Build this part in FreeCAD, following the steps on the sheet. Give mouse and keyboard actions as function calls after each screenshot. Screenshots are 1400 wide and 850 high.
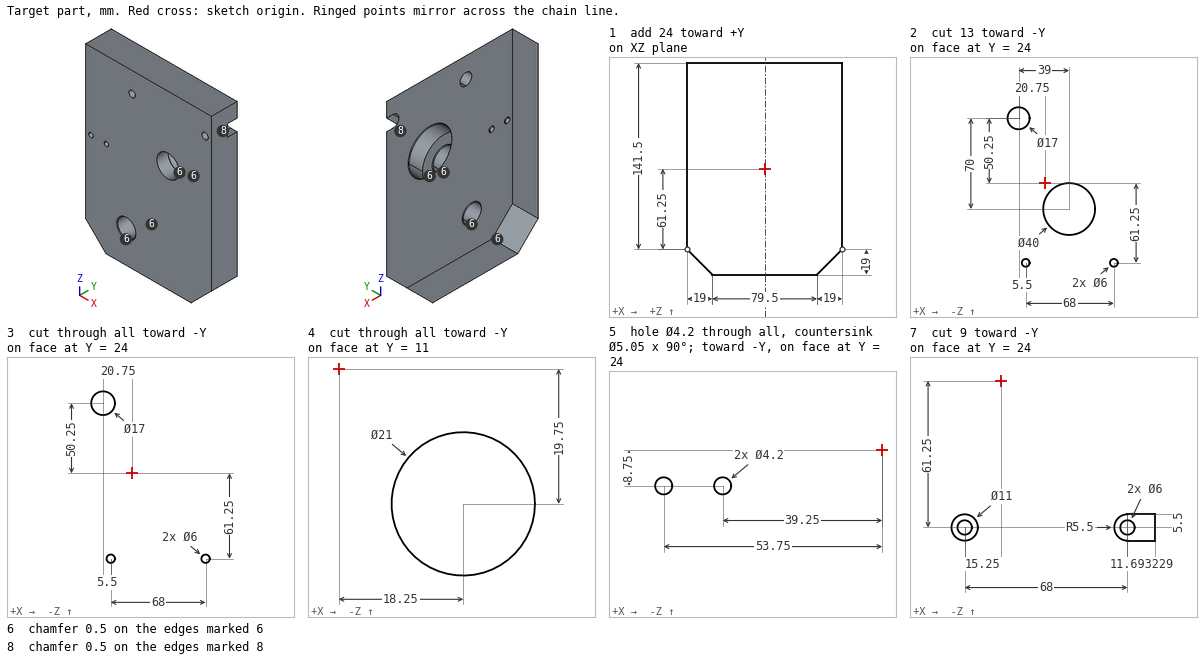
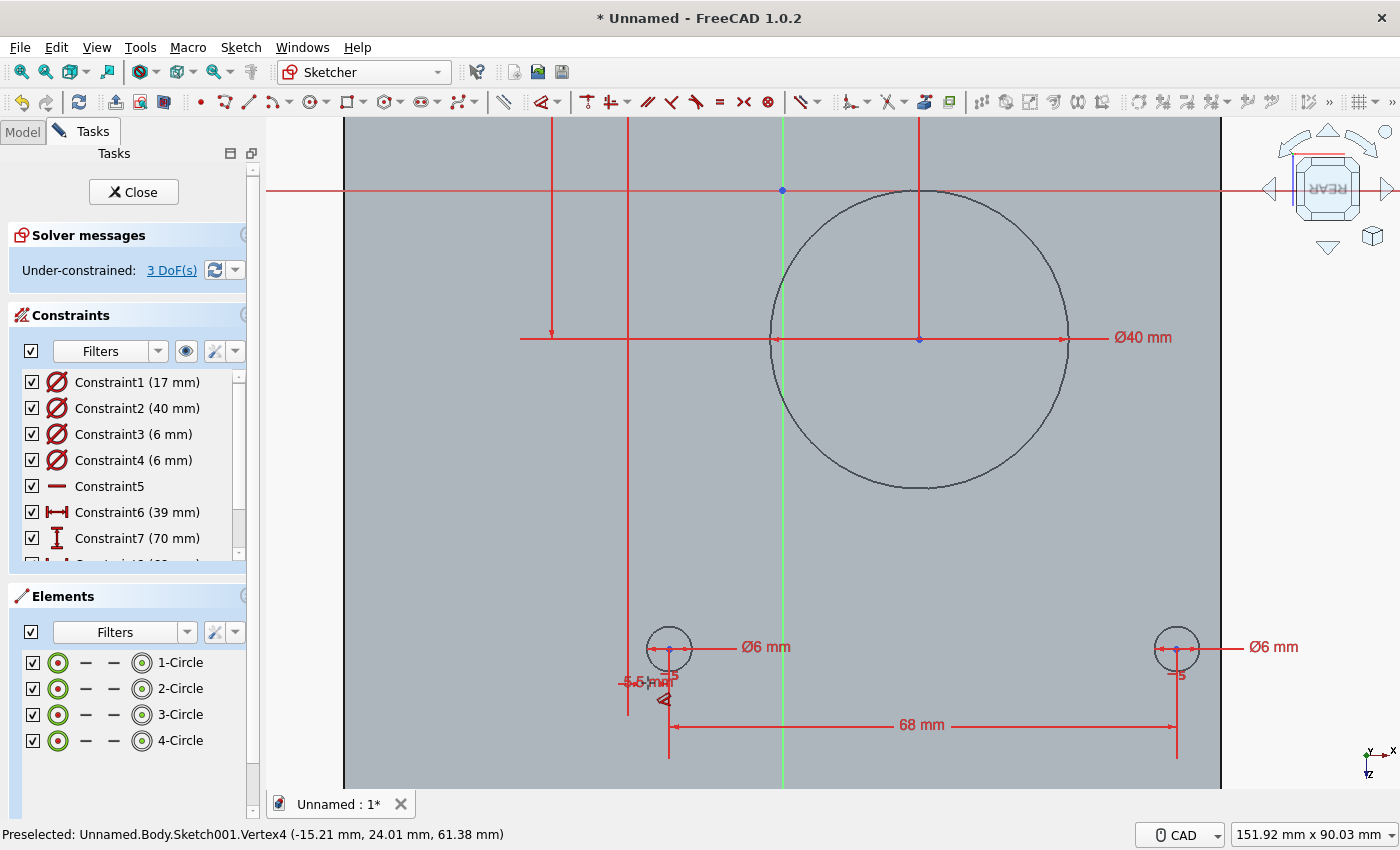
scroll(669, 650, down, 4)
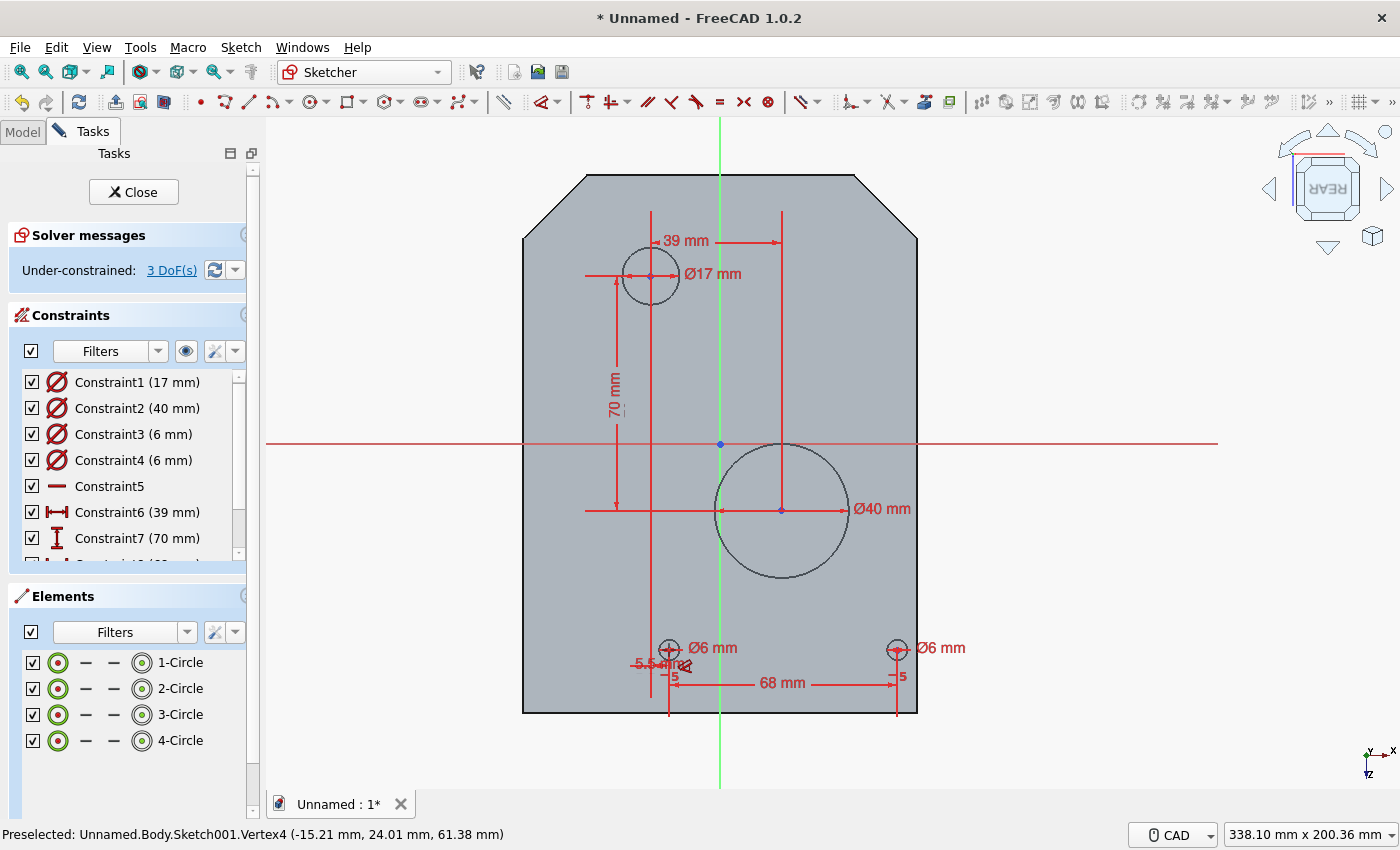
click(651, 276)
click(686, 478)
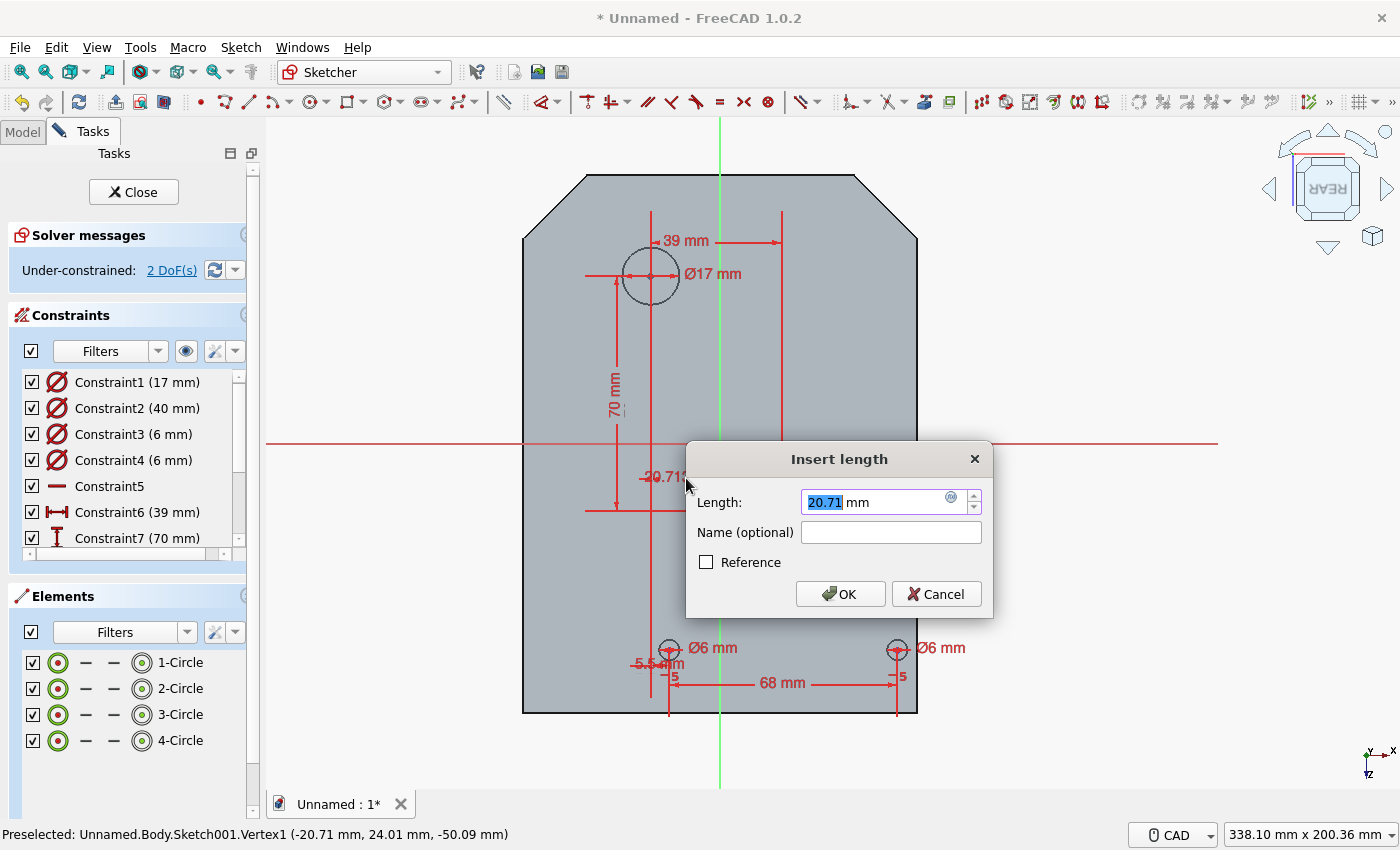
text(20.75)
key(Return)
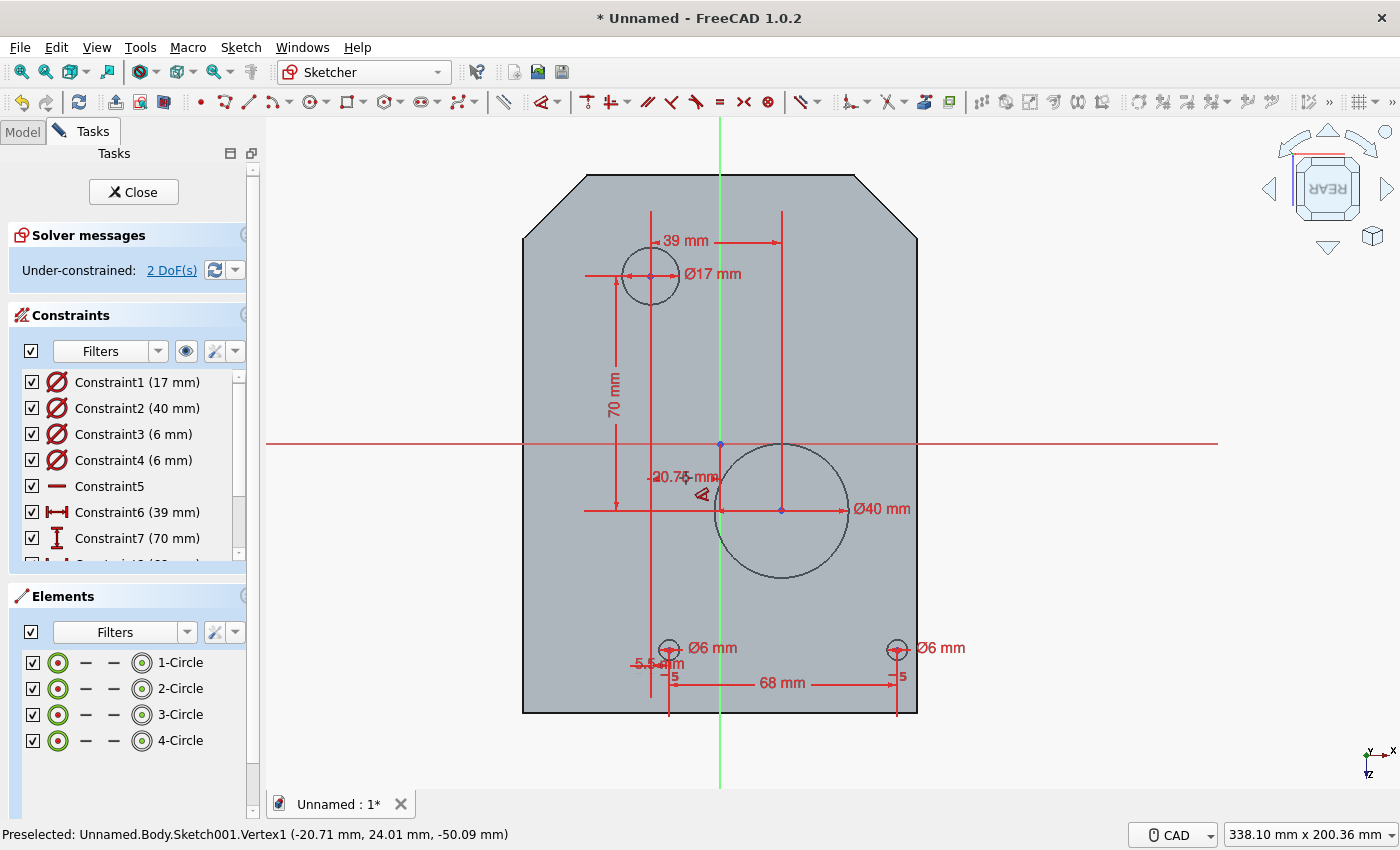
click(651, 276)
click(617, 360)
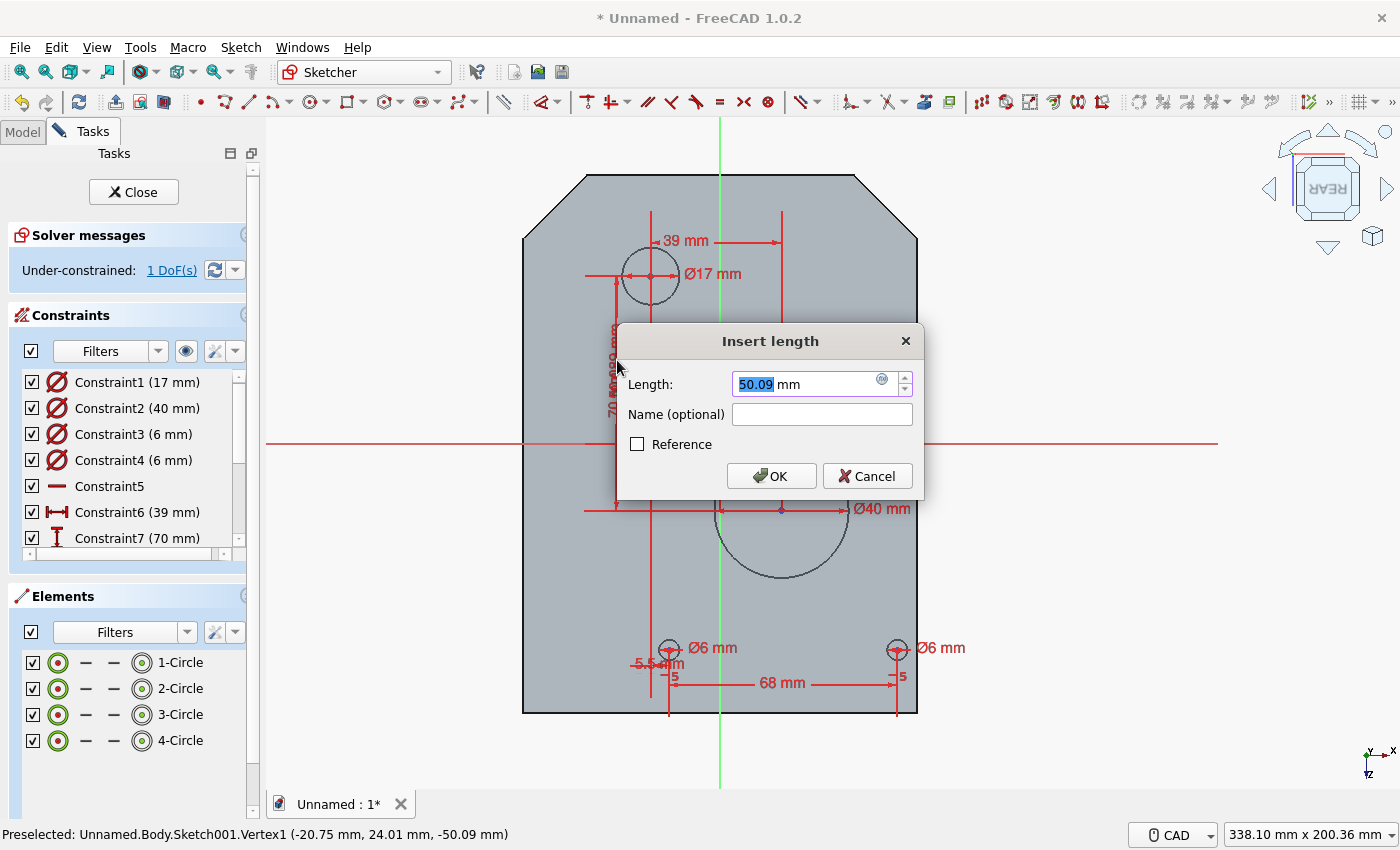
text(50.25)
key(Return)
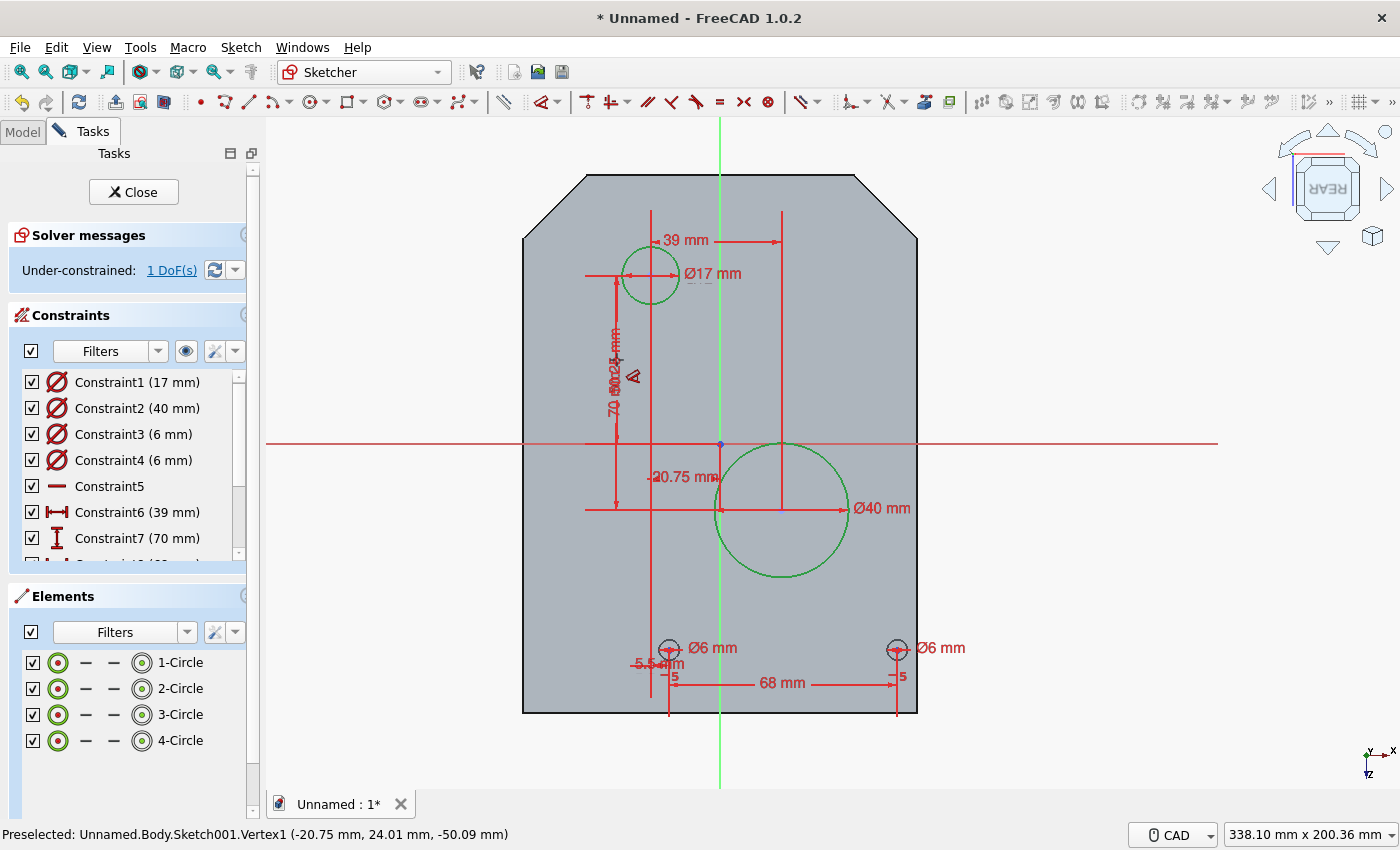
click(897, 650)
click(931, 547)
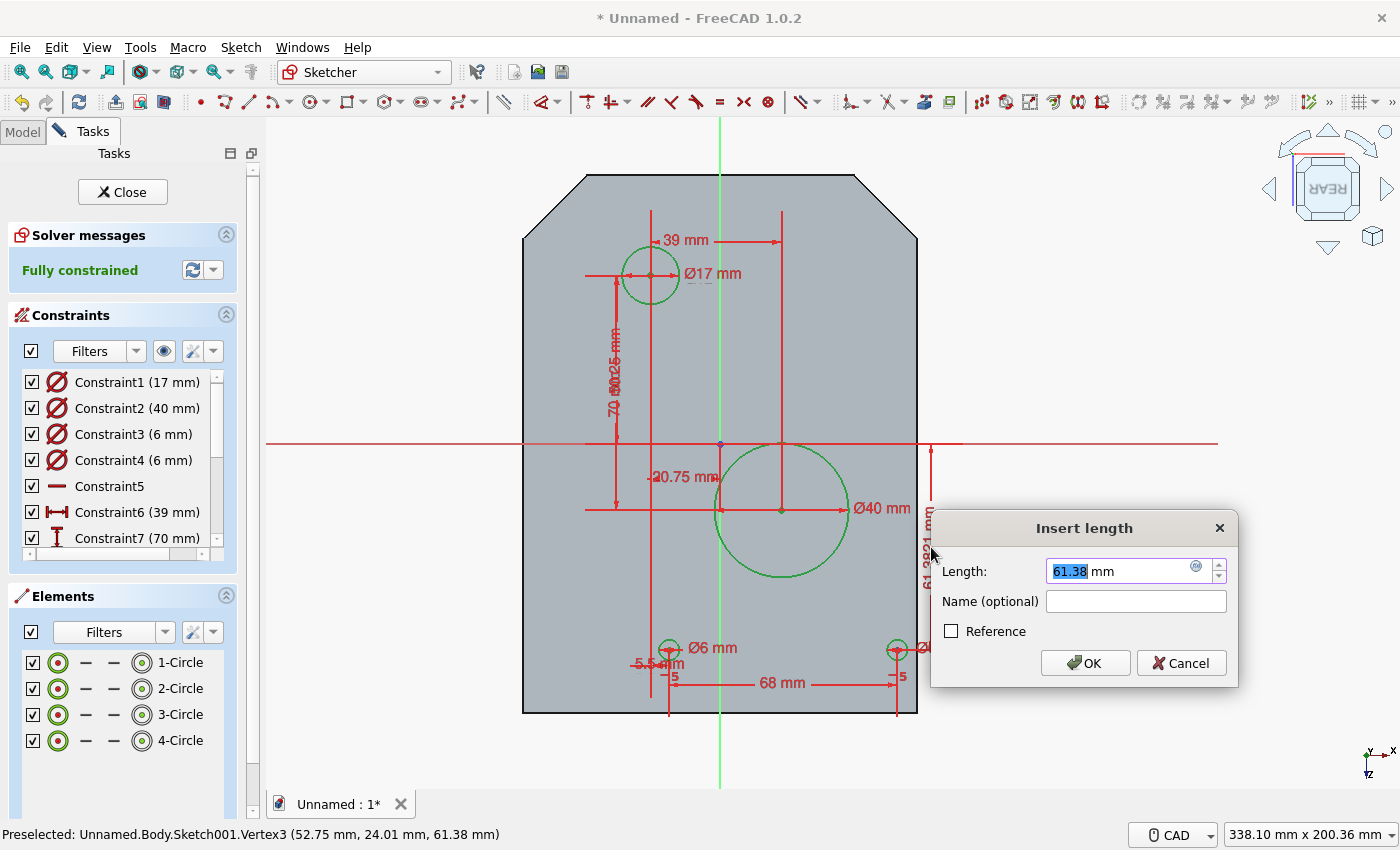
text(61.25)
key(Return)
key(Escape)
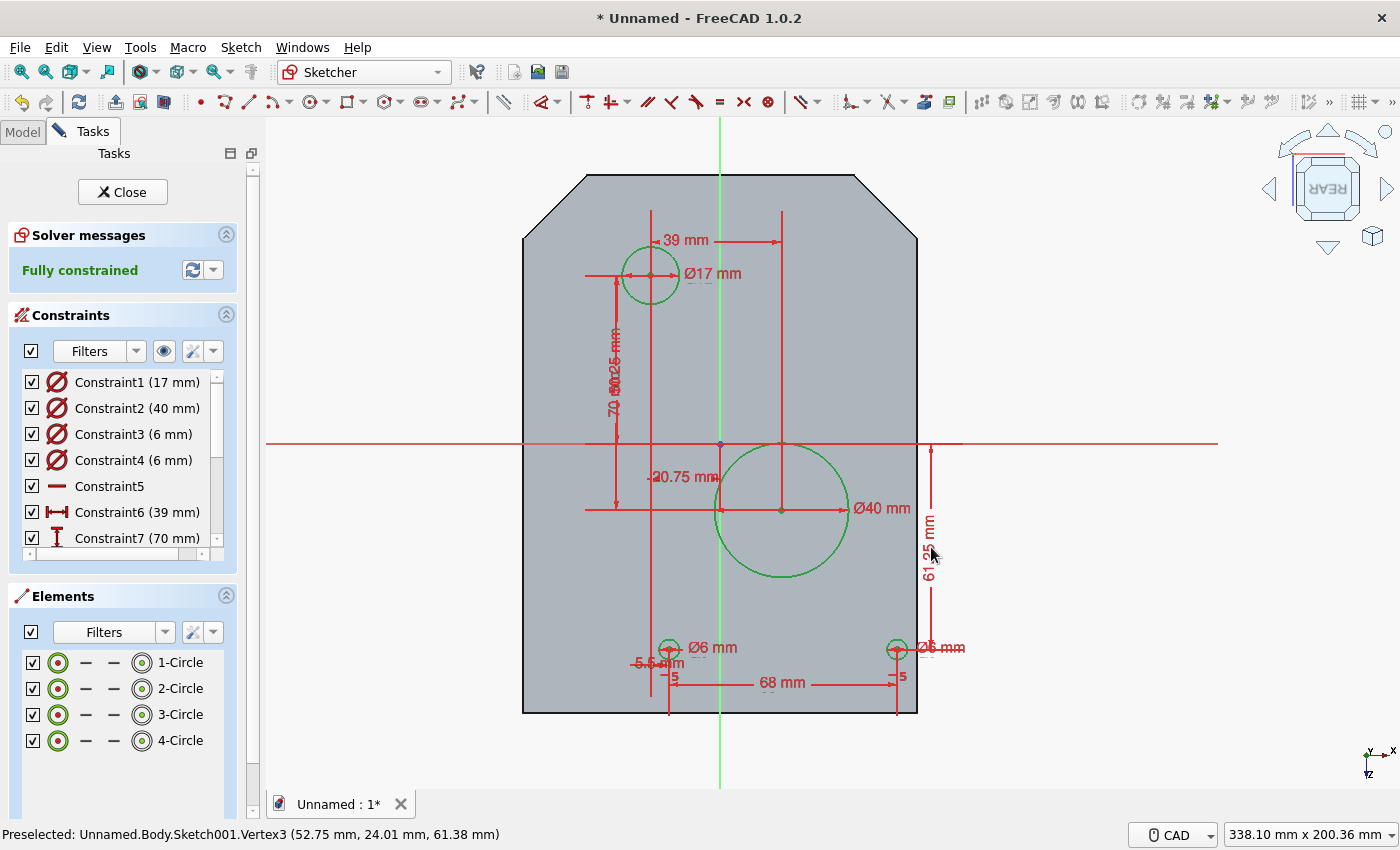
click(123, 192)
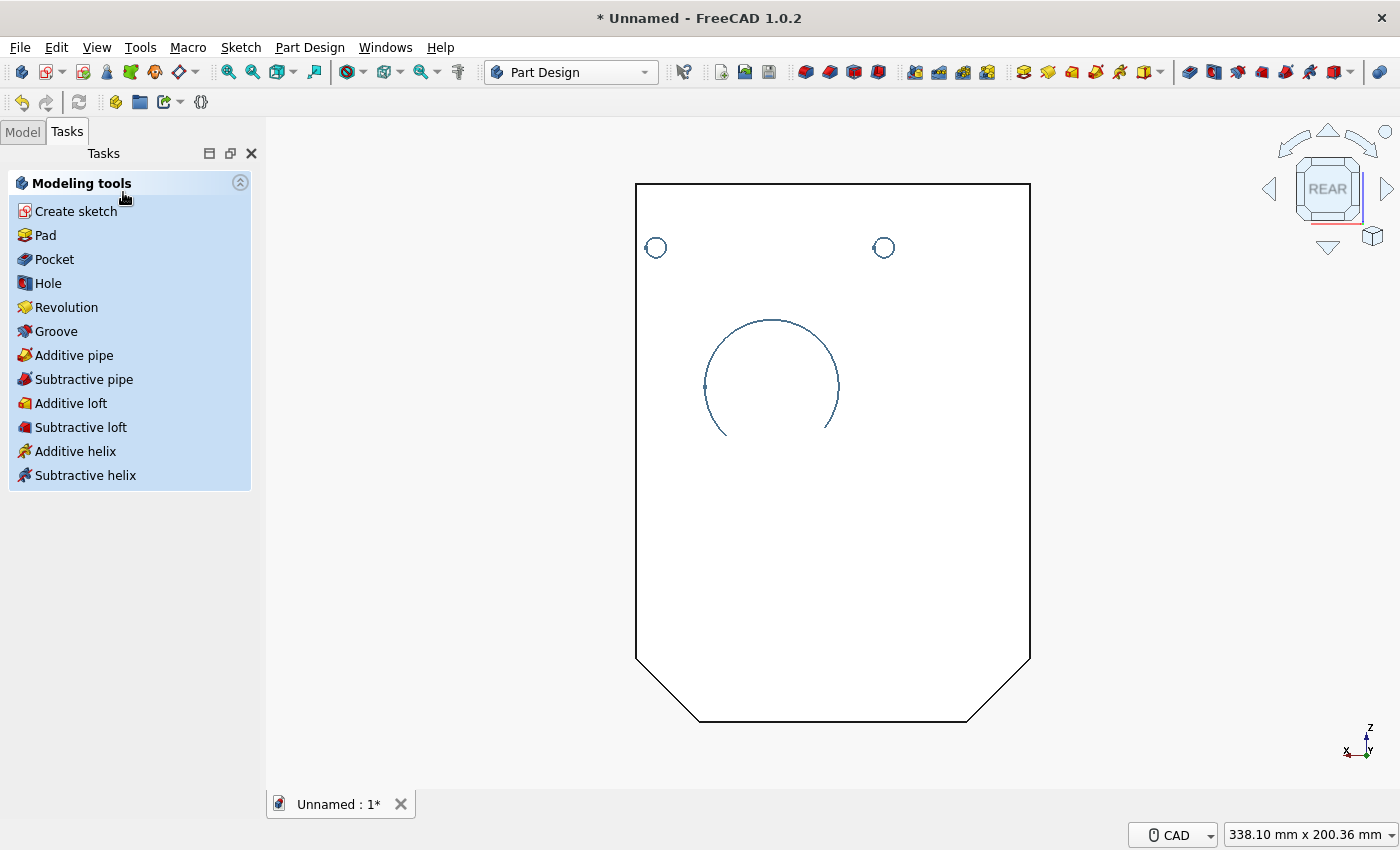
click(1190, 72)